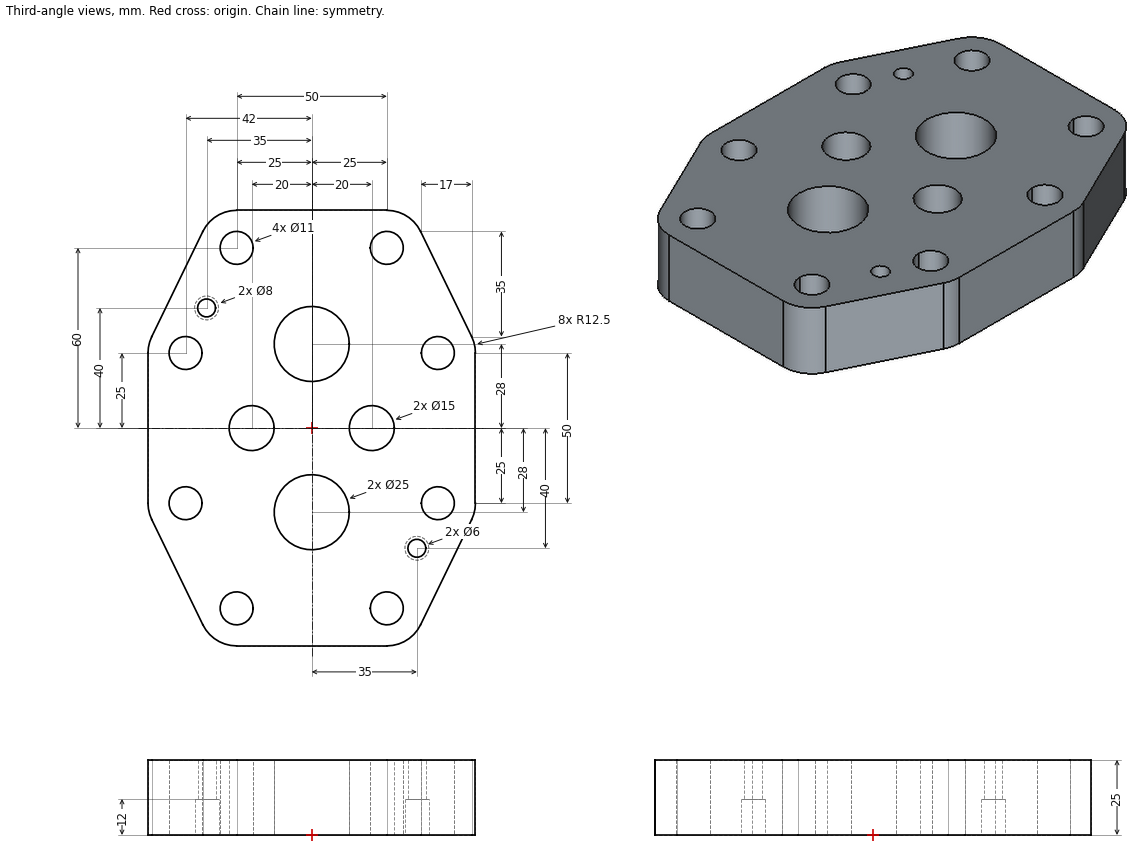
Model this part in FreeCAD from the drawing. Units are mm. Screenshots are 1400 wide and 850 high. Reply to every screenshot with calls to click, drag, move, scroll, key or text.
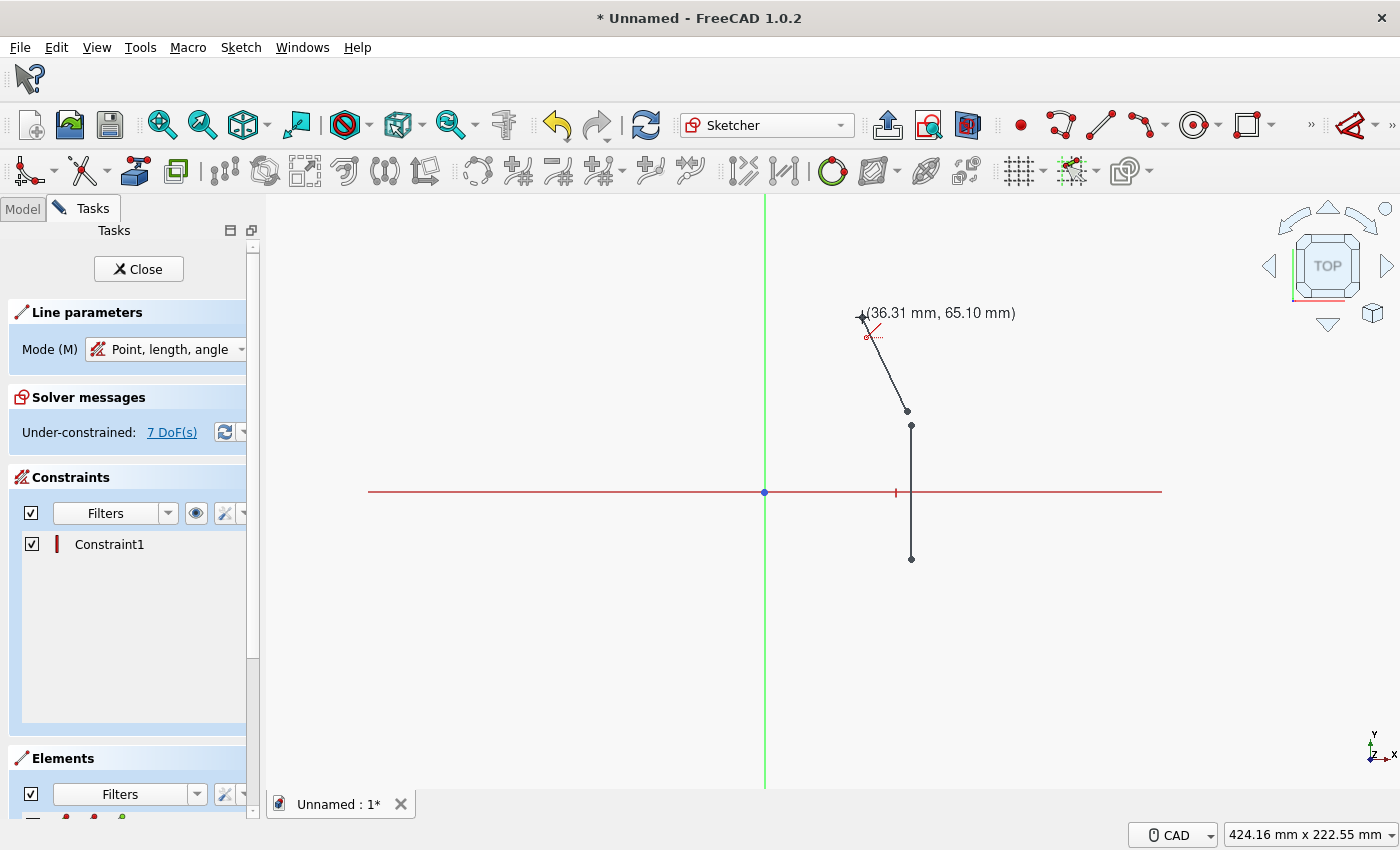
click(832, 298)
click(698, 298)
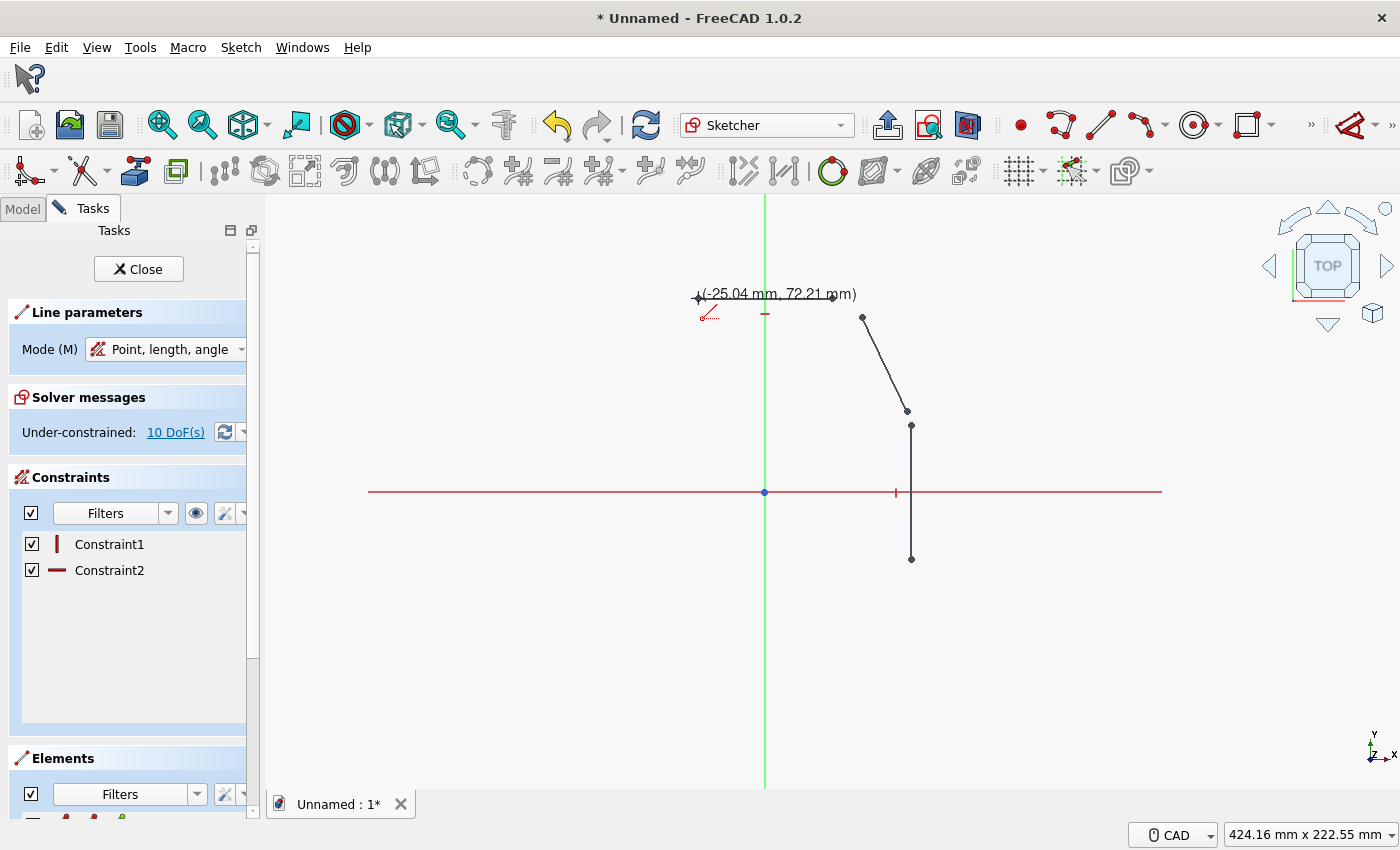
click(668, 317)
click(623, 411)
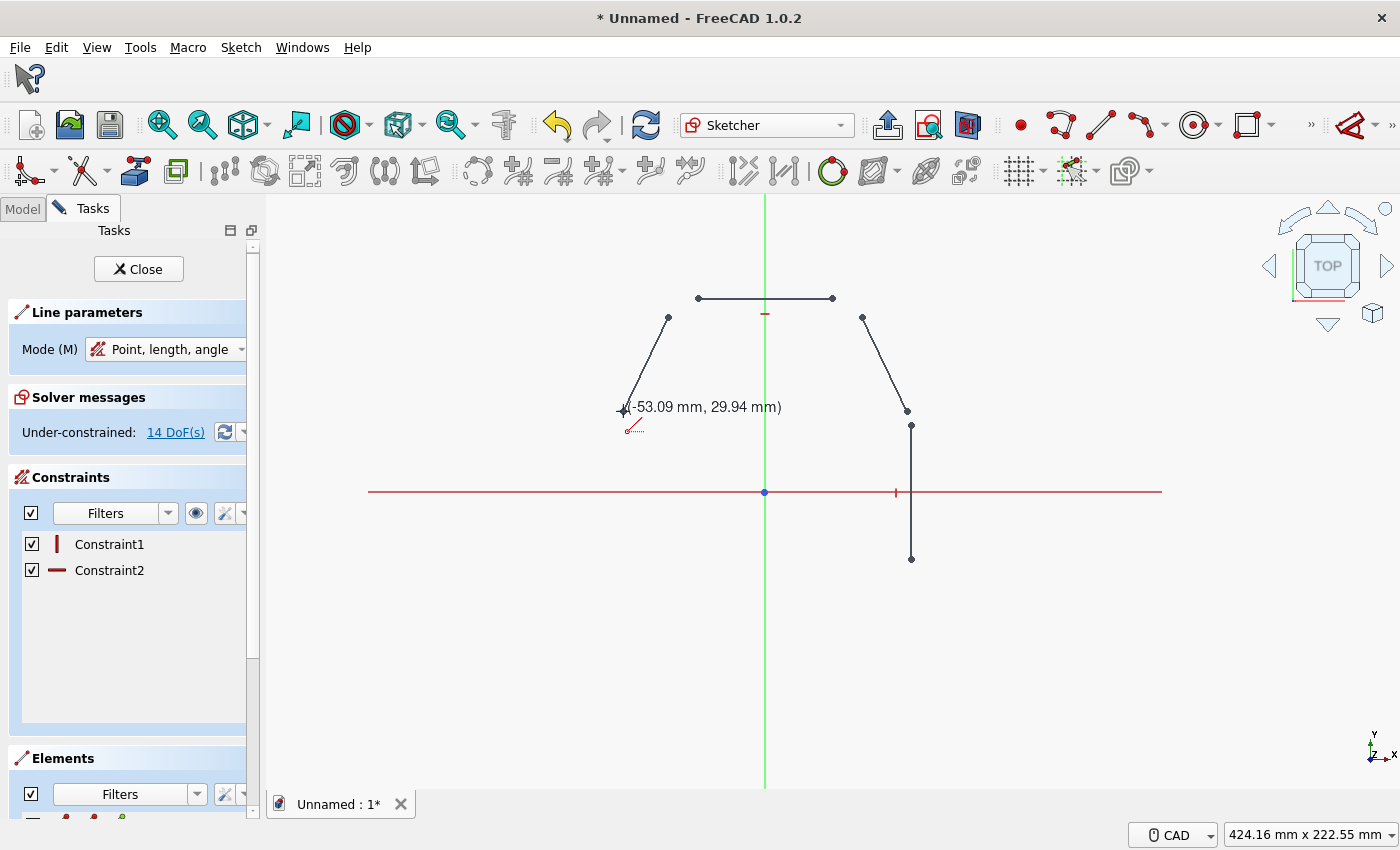
click(619, 425)
click(619, 559)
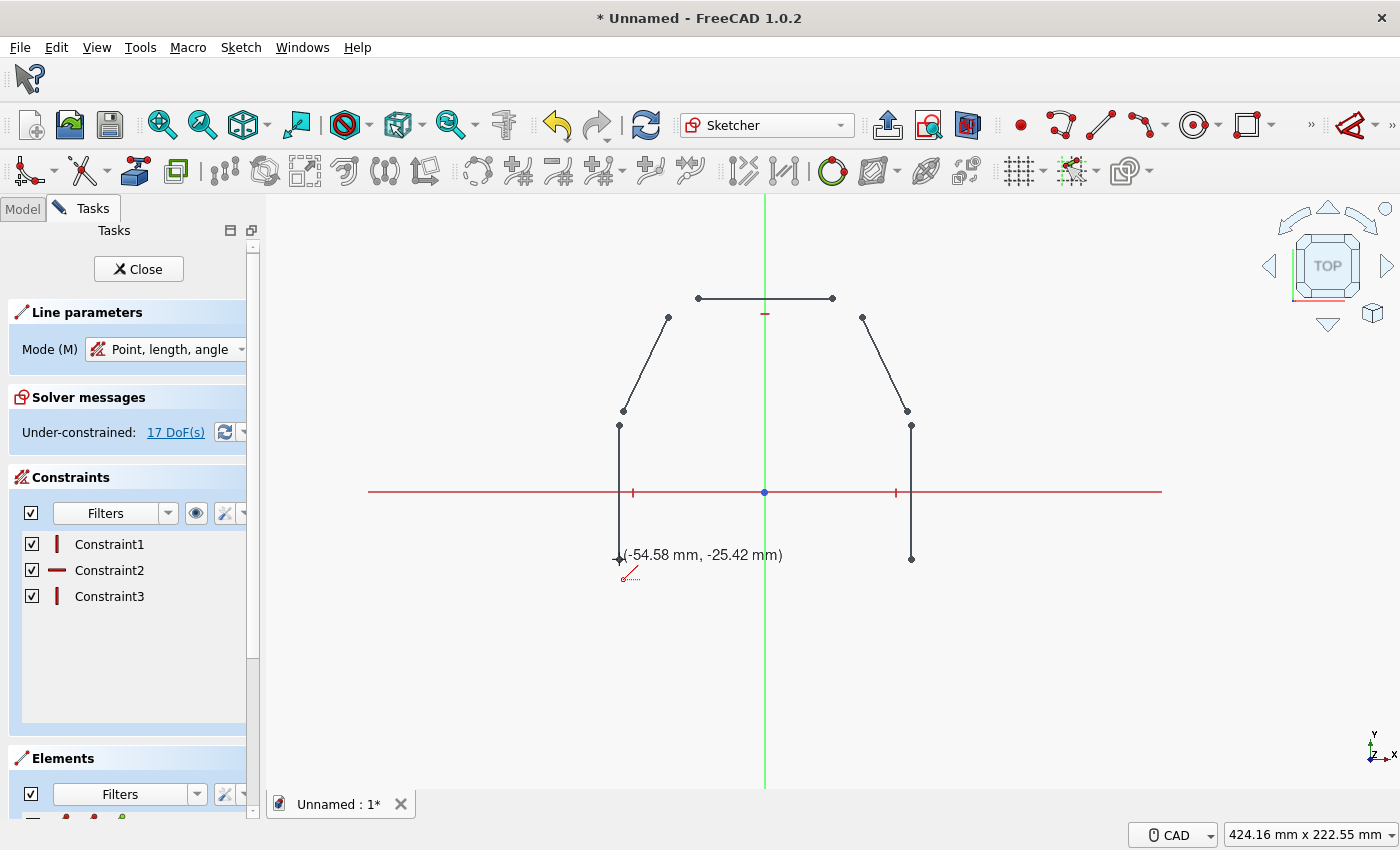
click(623, 573)
click(668, 667)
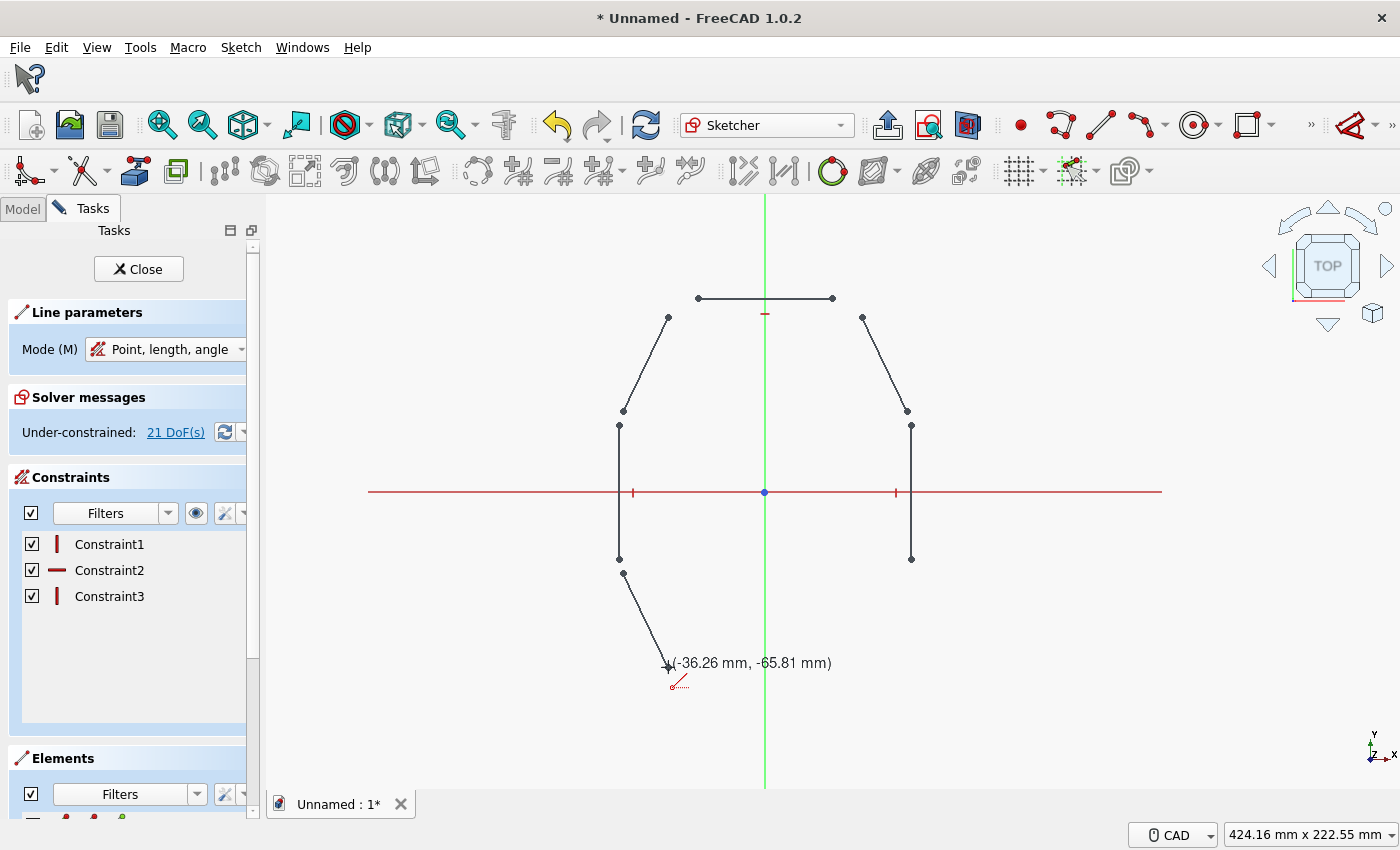
click(698, 686)
click(832, 686)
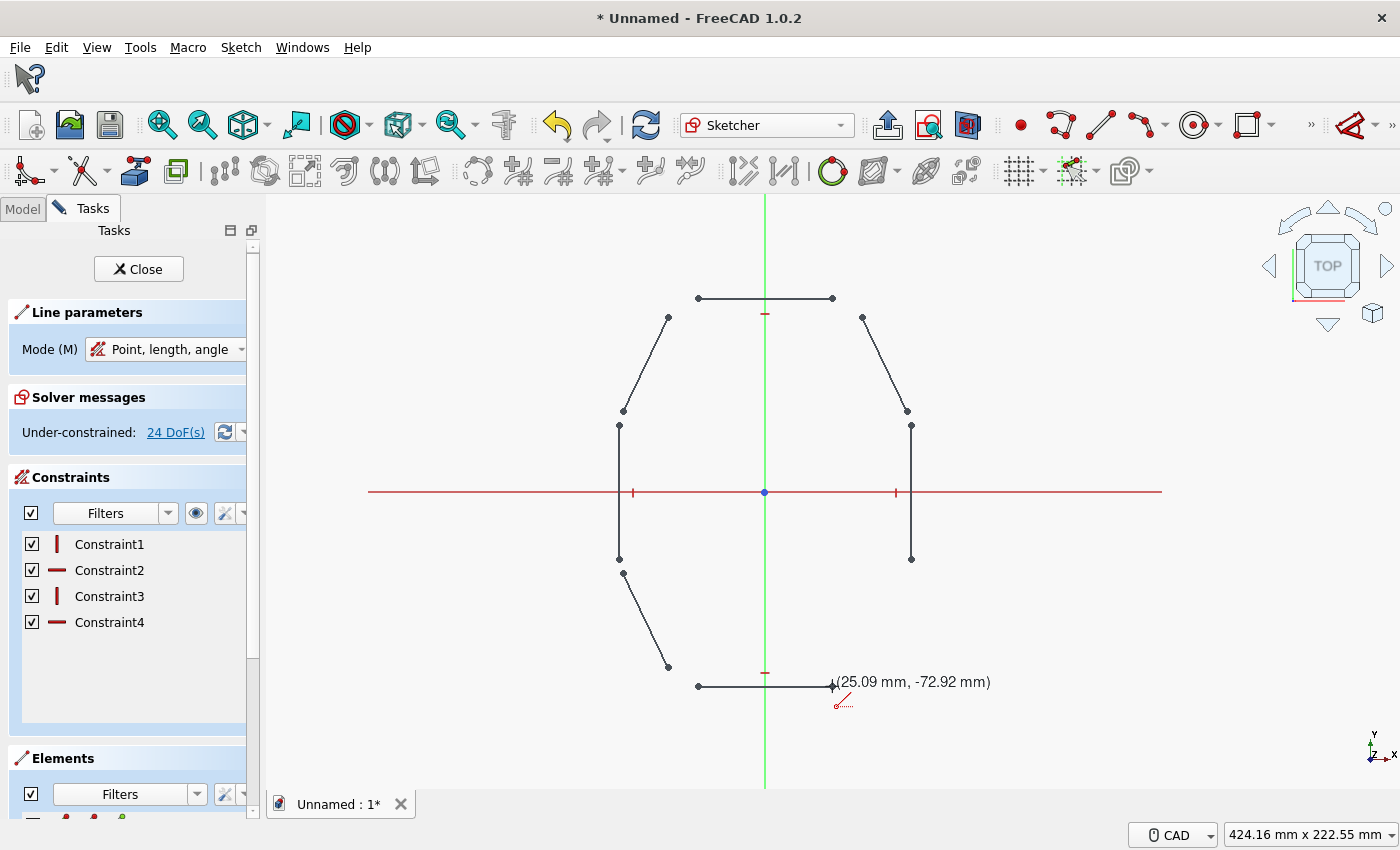
click(862, 667)
click(907, 573)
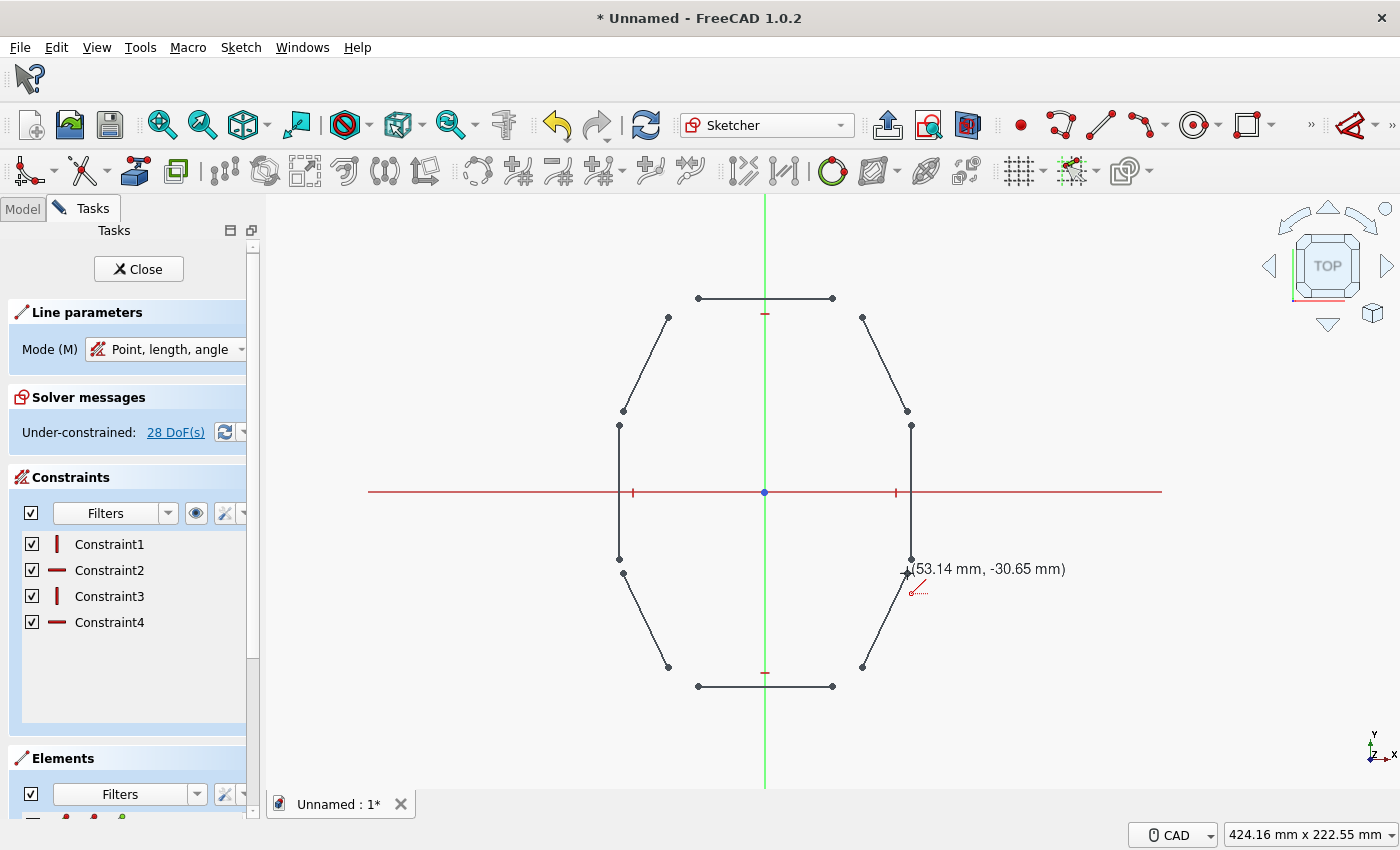
key(g)
key(3)
key(a)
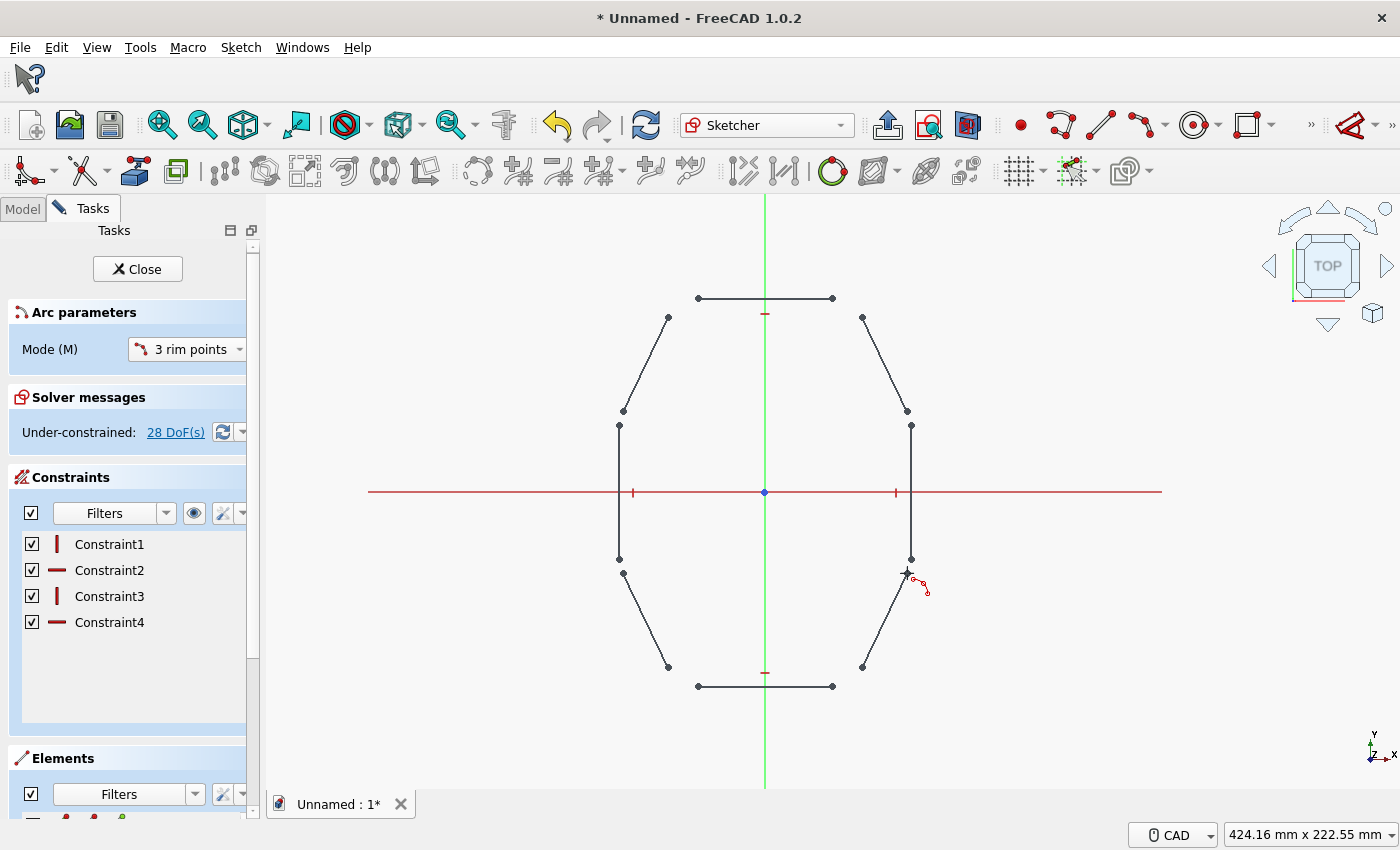
click(911, 426)
click(907, 412)